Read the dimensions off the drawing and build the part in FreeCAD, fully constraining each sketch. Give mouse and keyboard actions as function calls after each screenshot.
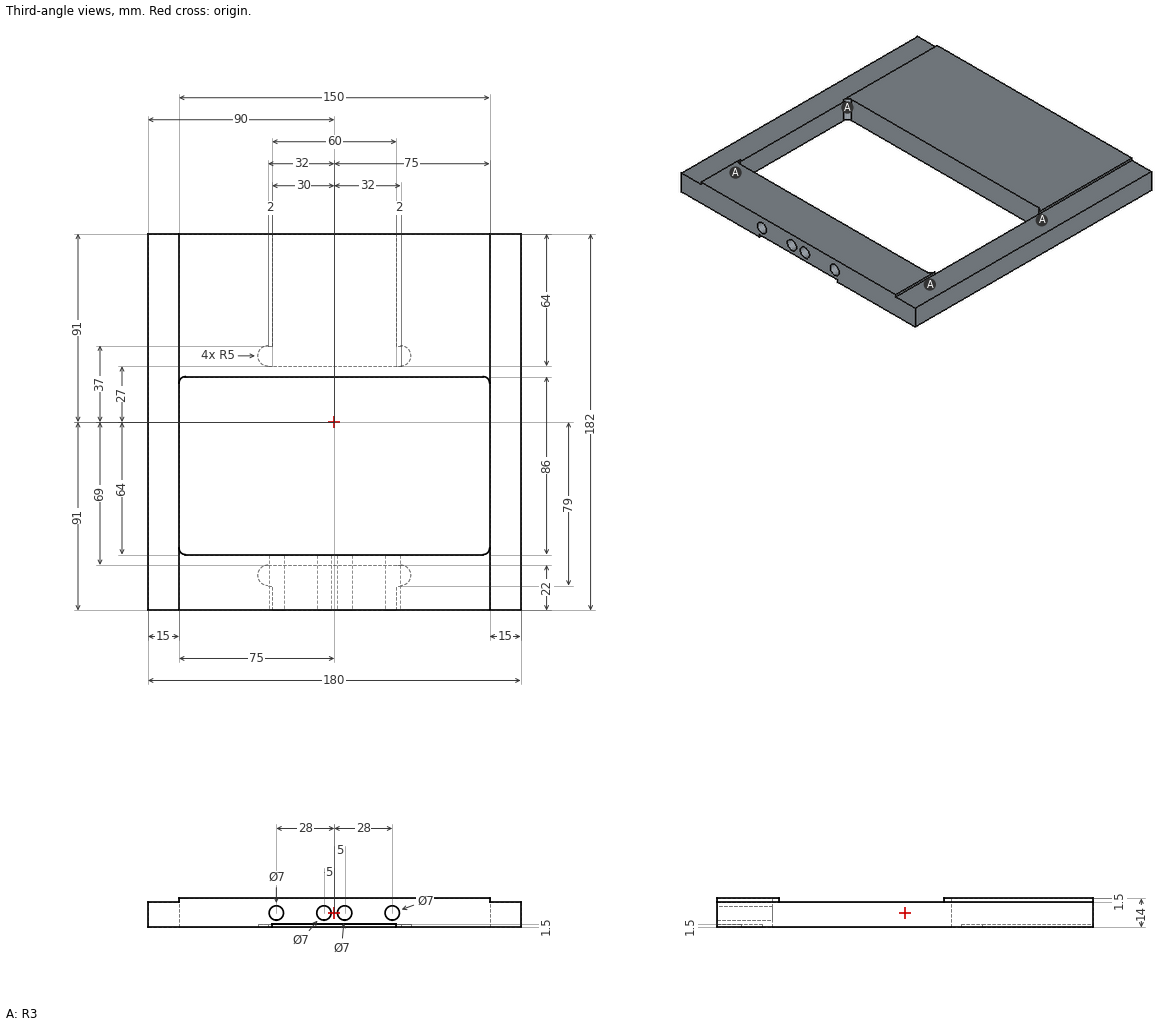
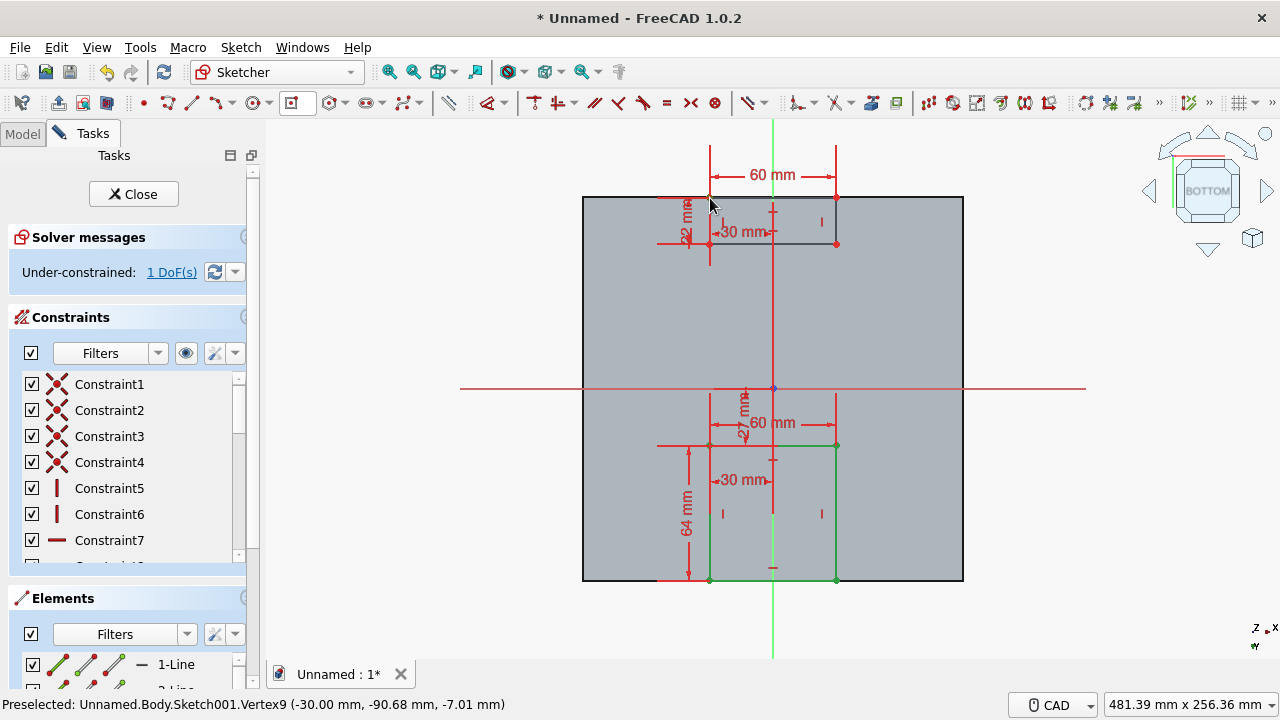
click(506, 104)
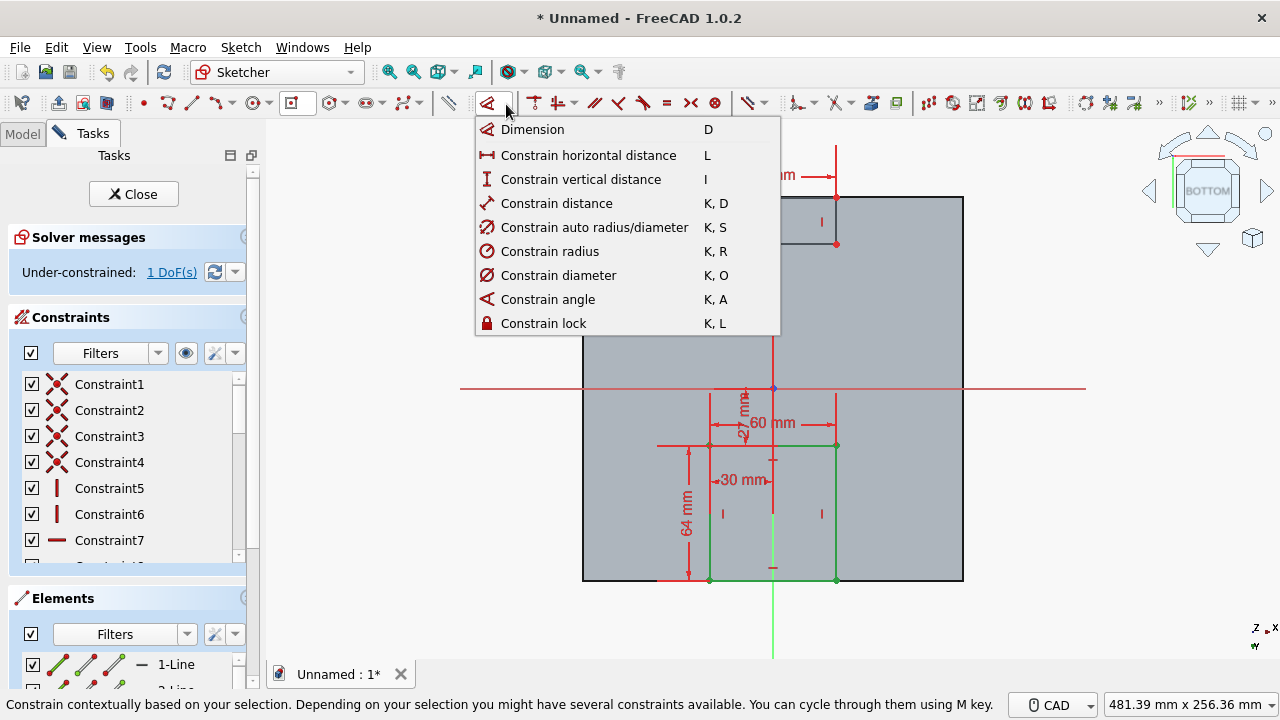
click(628, 179)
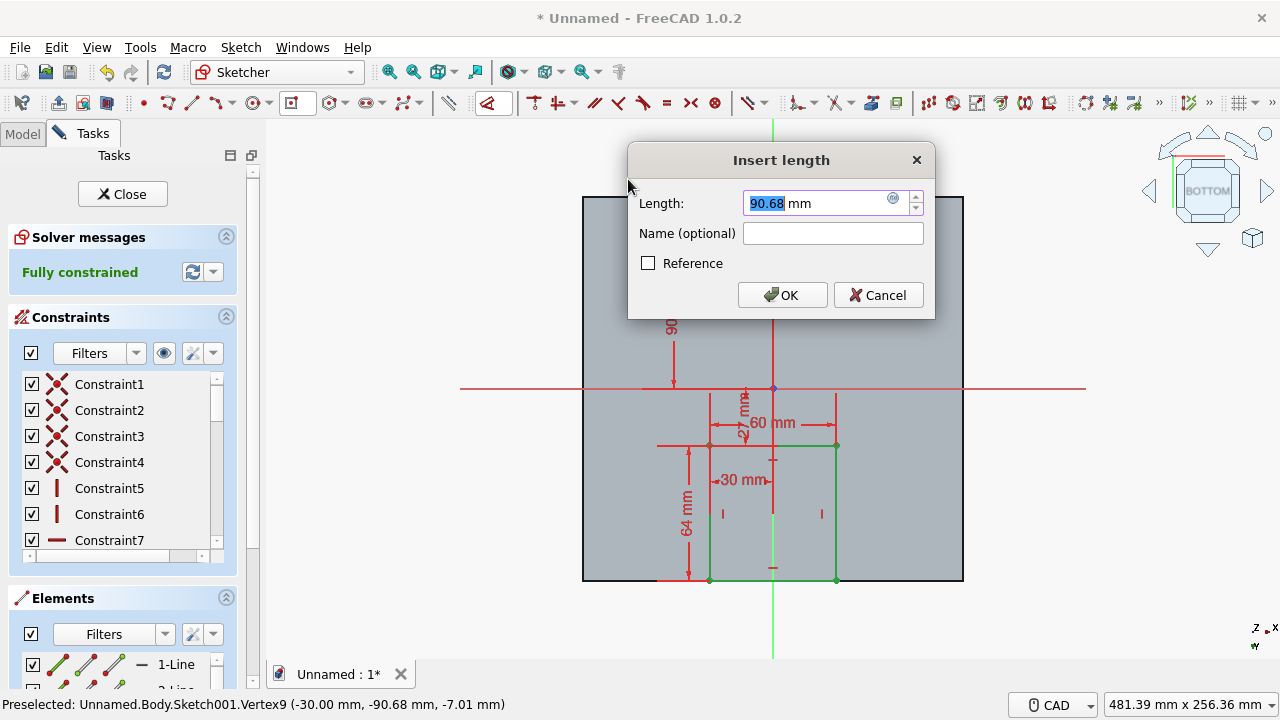
text(91)
key(Return)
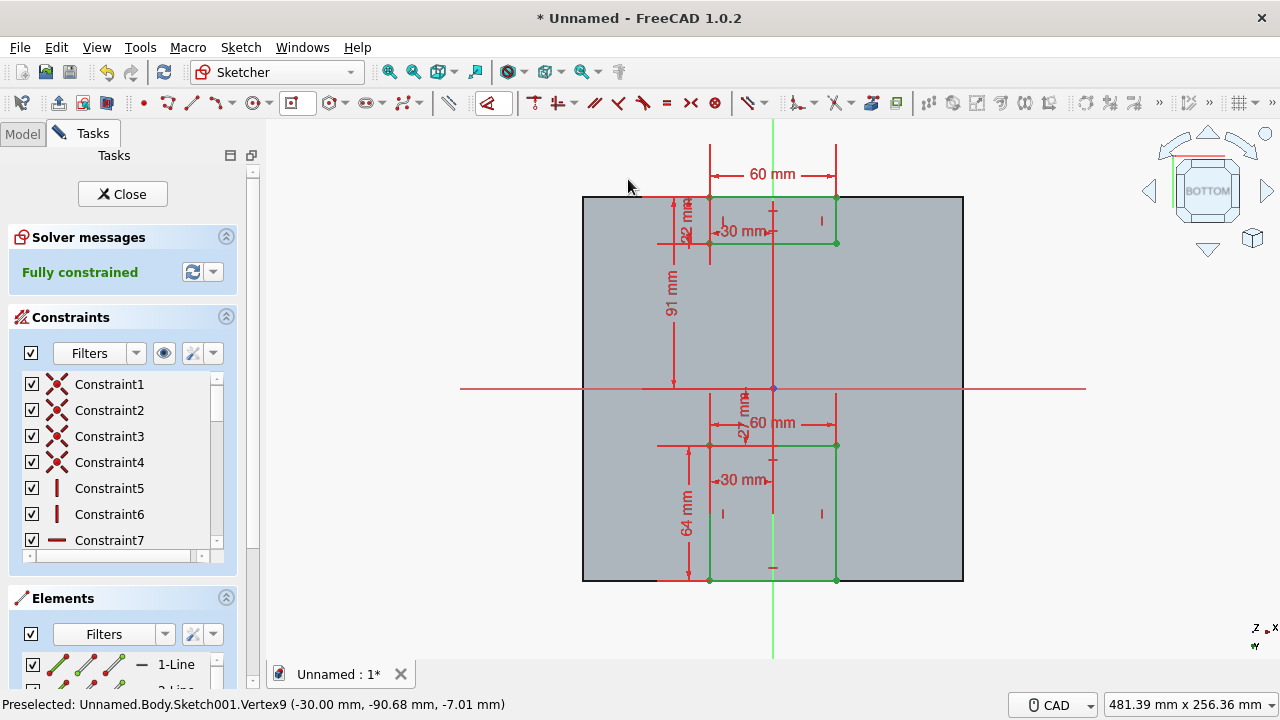
click(123, 194)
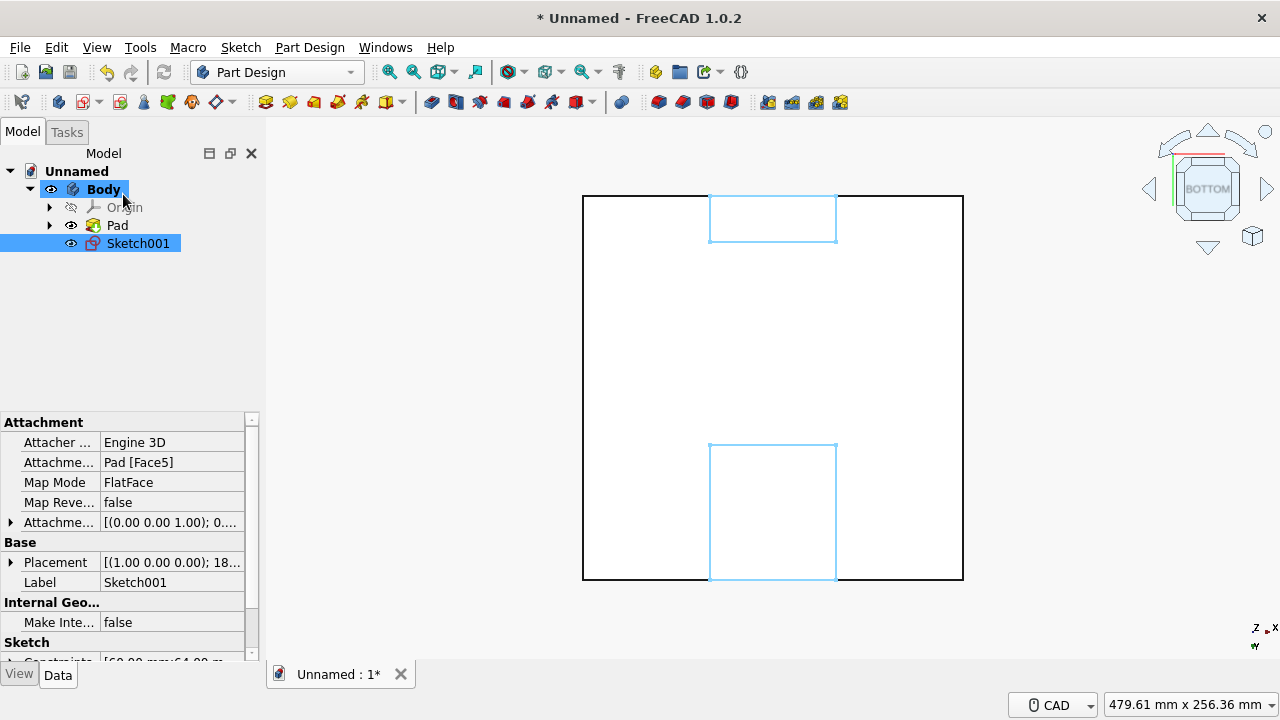
click(432, 102)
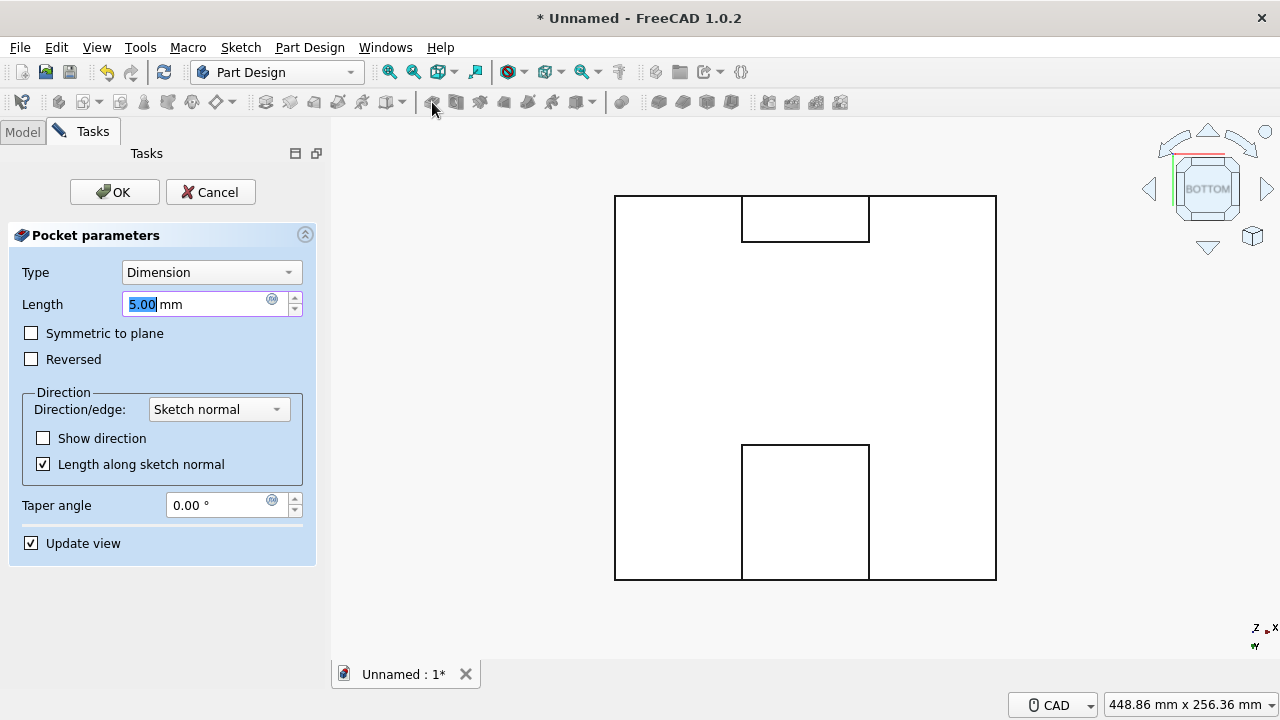
text(1.5)
key(Tab)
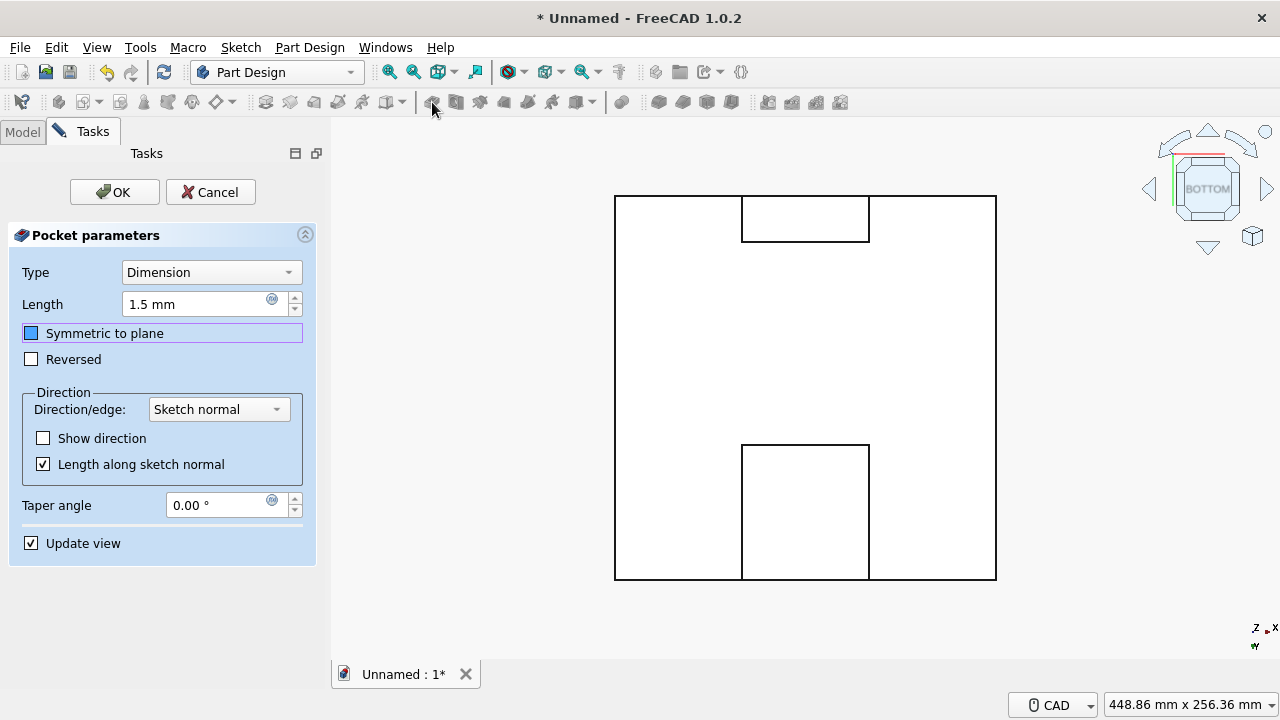
click(115, 192)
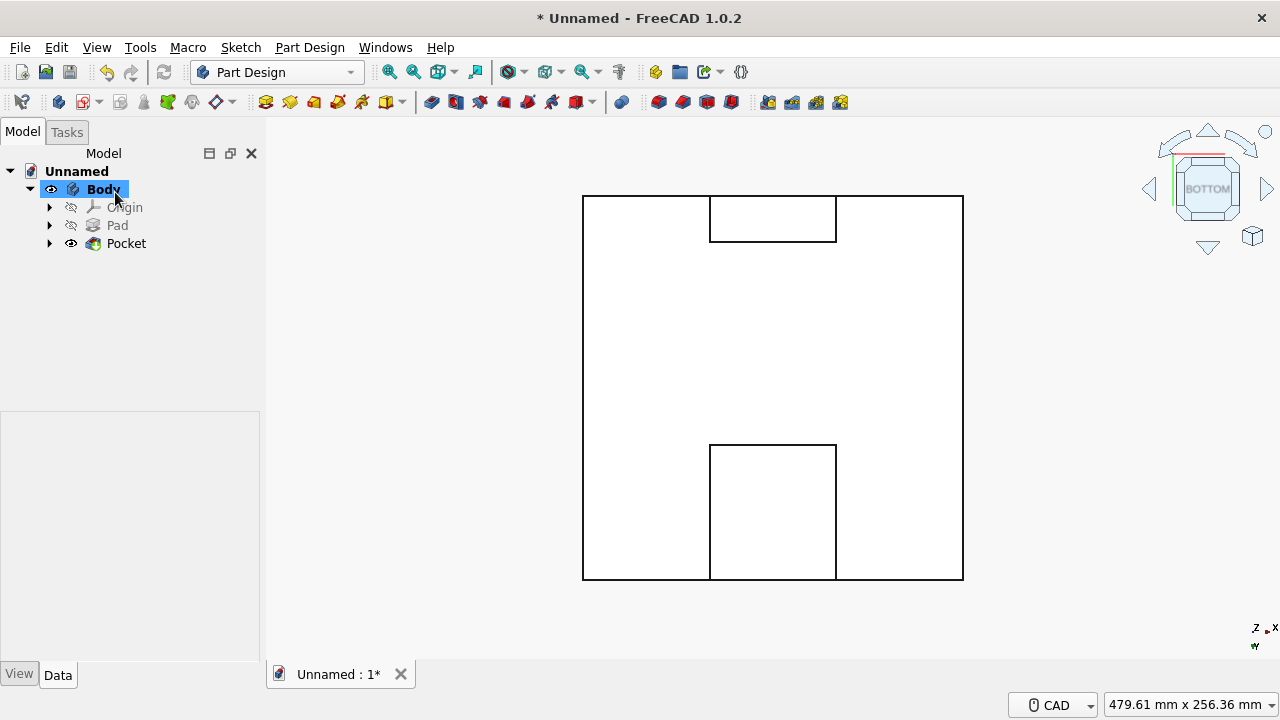
click(827, 332)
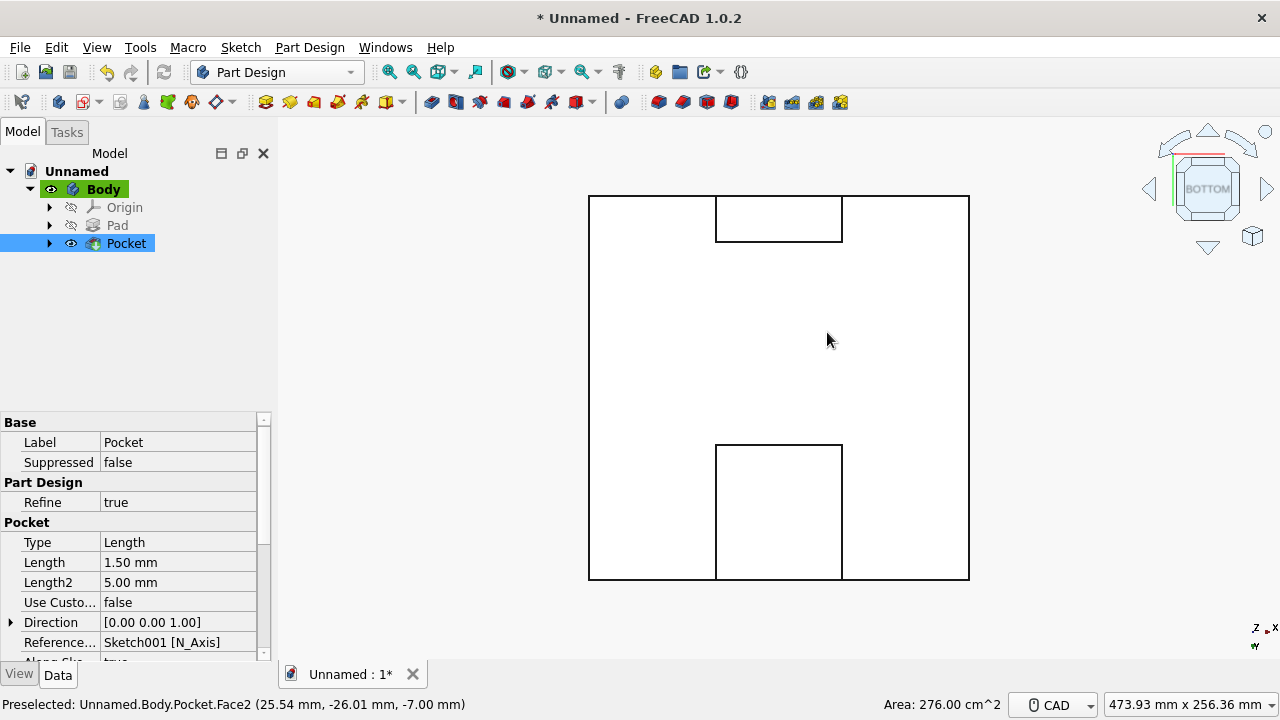
click(84, 102)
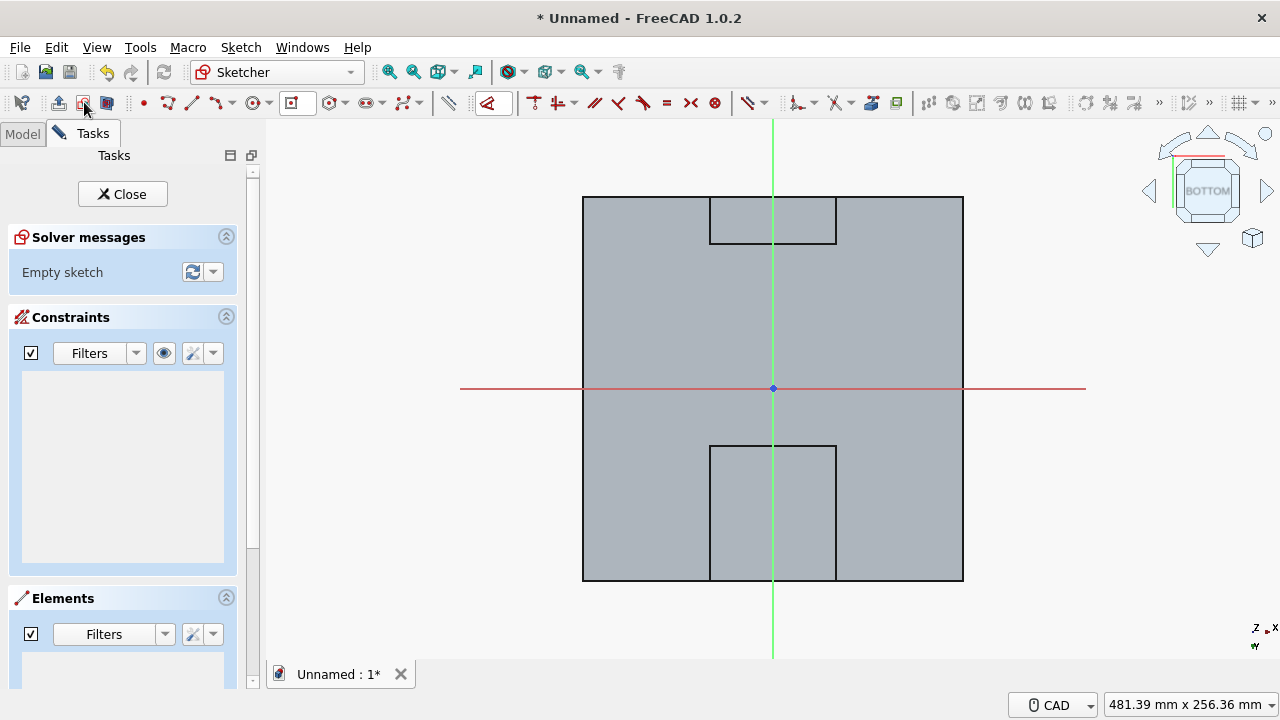
scroll(912, 255, up, 2)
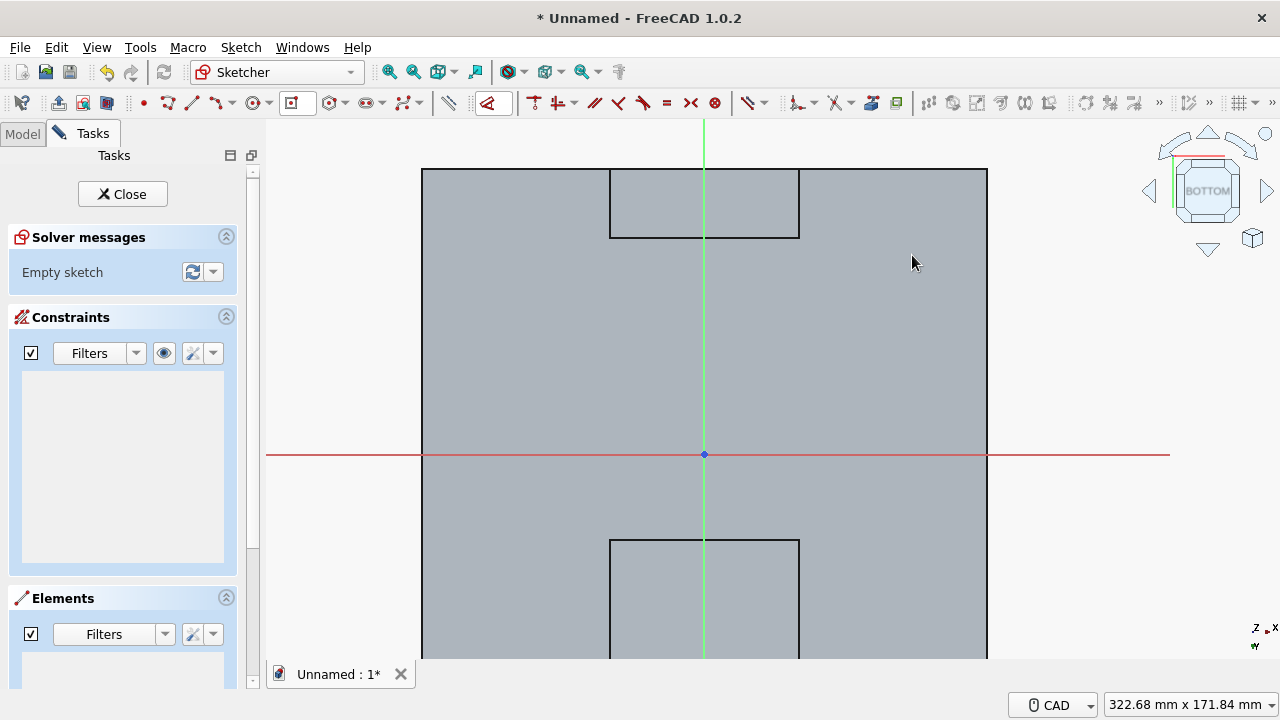
click(168, 104)